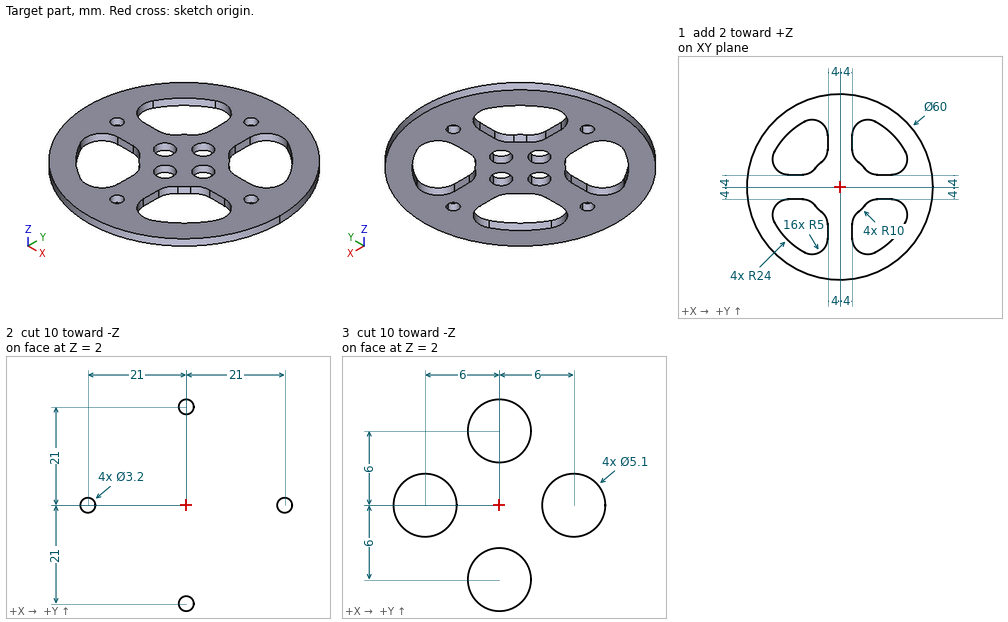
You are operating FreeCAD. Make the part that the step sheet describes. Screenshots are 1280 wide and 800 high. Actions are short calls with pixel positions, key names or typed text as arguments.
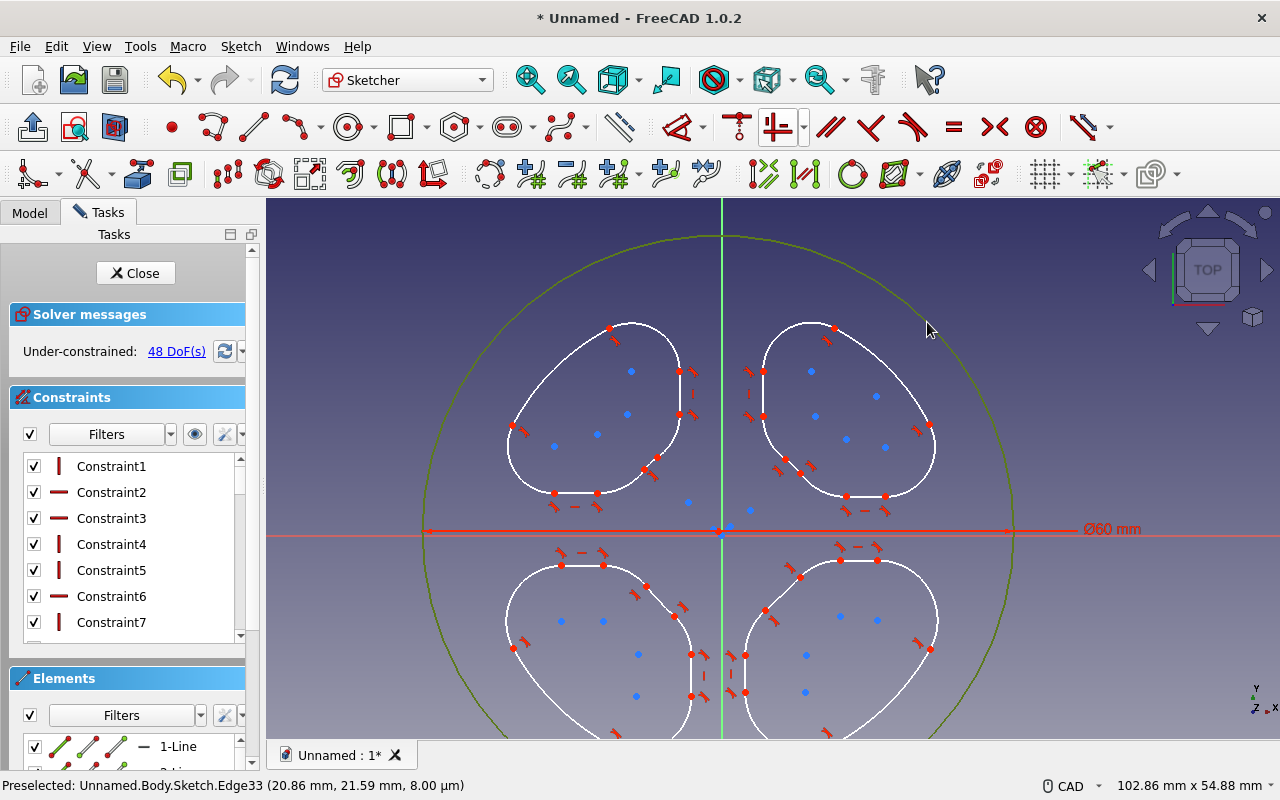
click(536, 683)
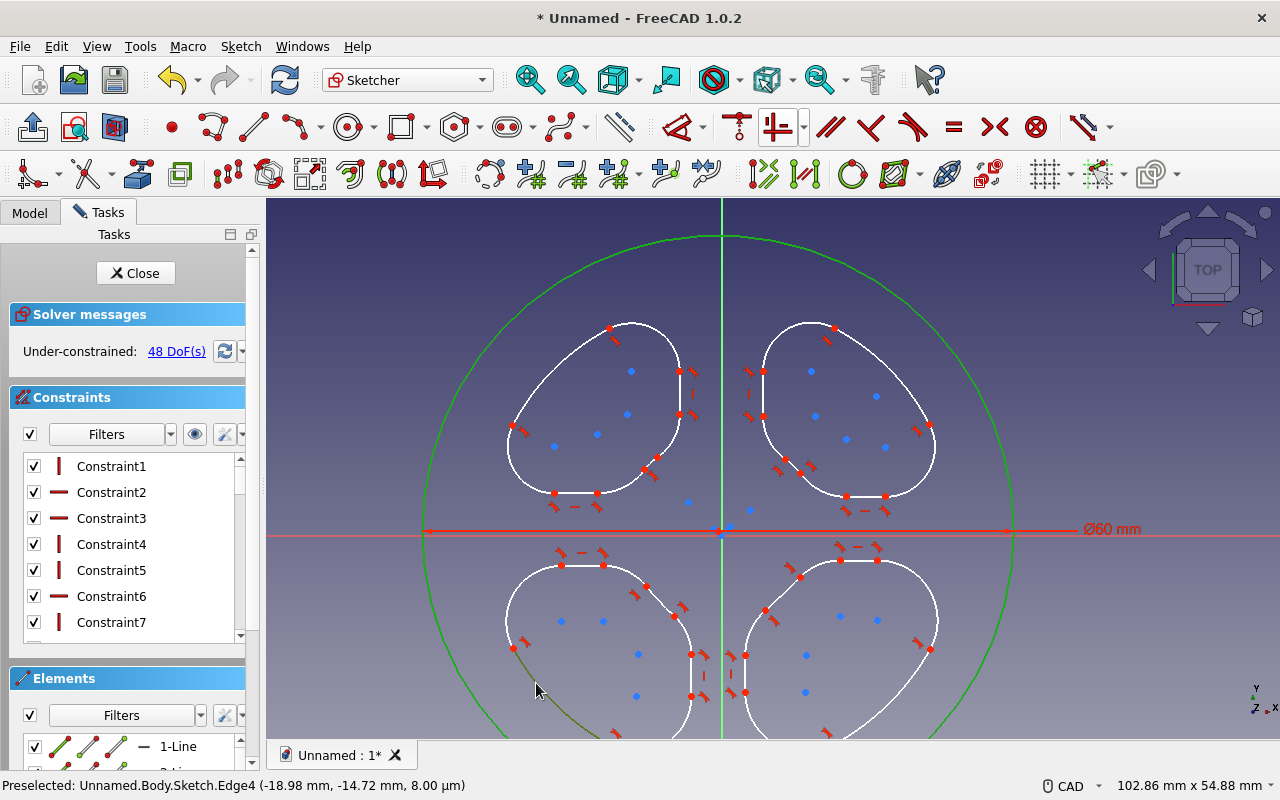
click(737, 128)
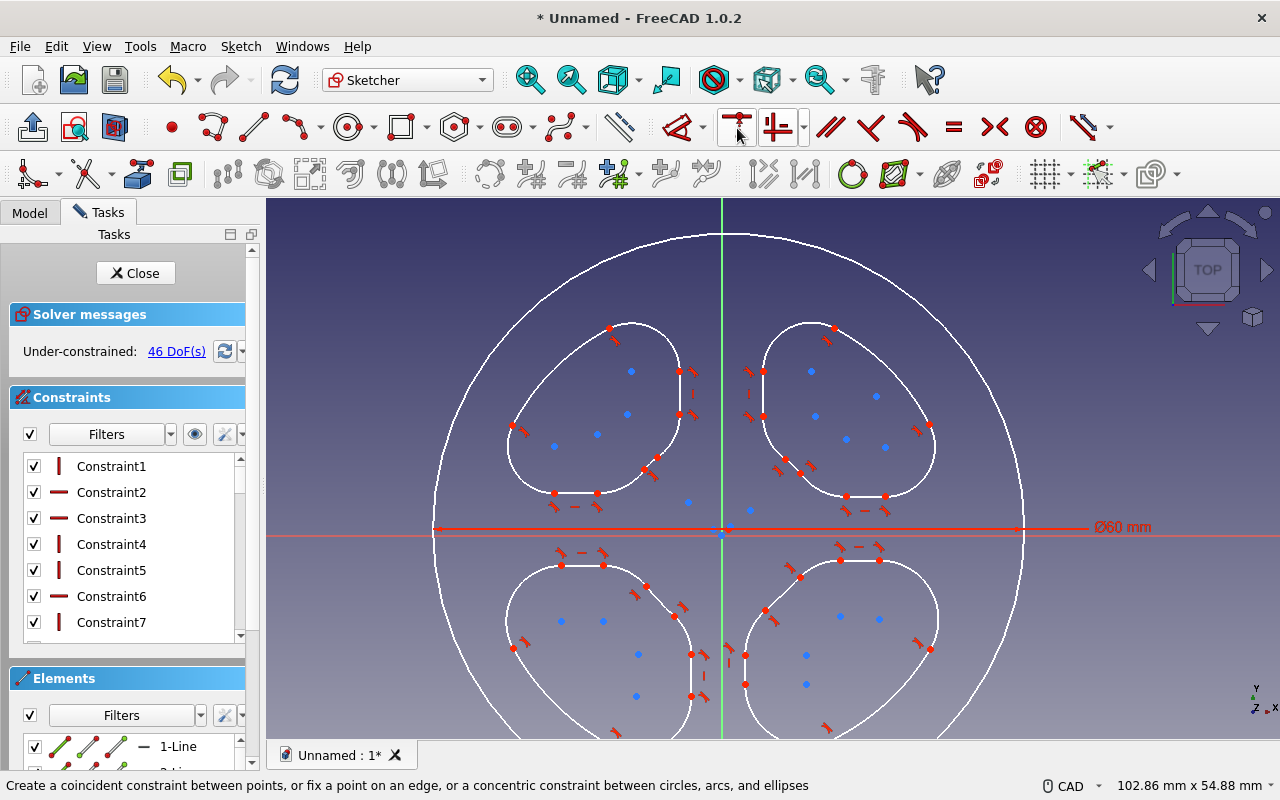
click(937, 320)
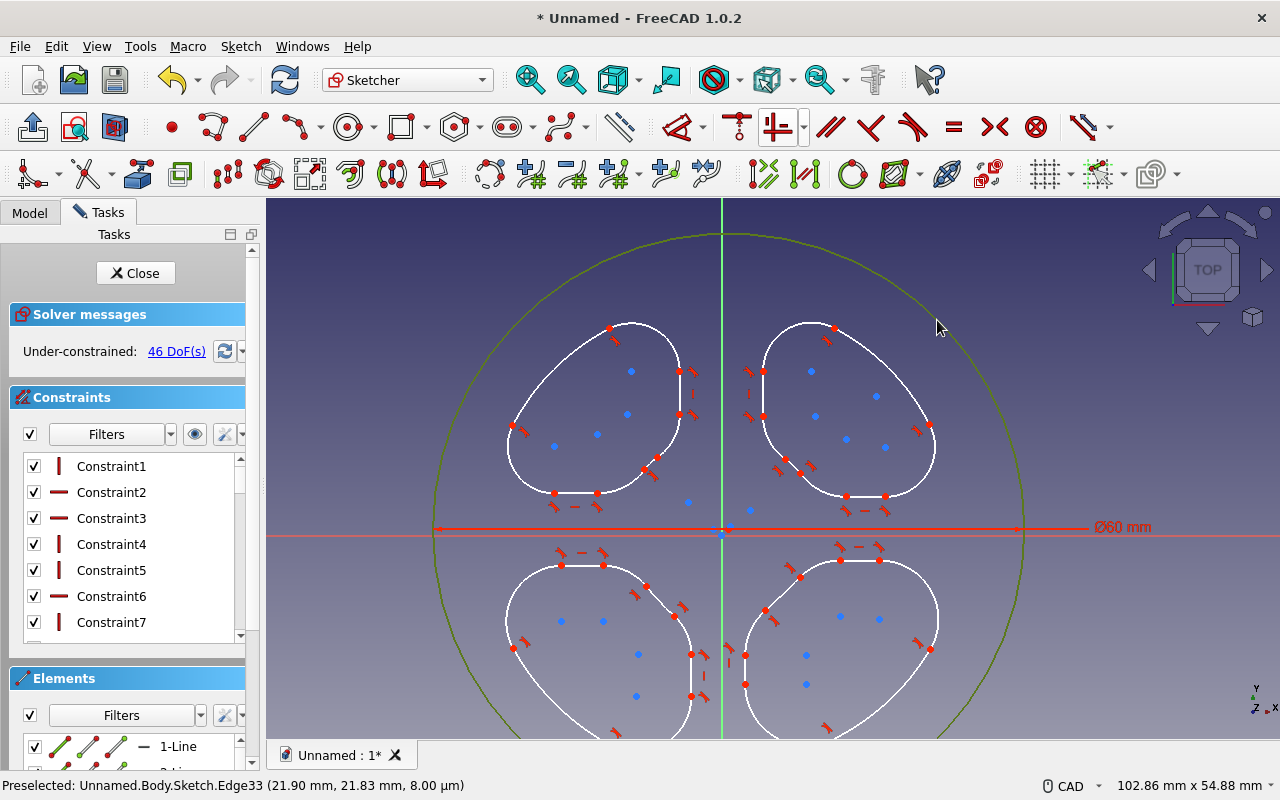
click(654, 596)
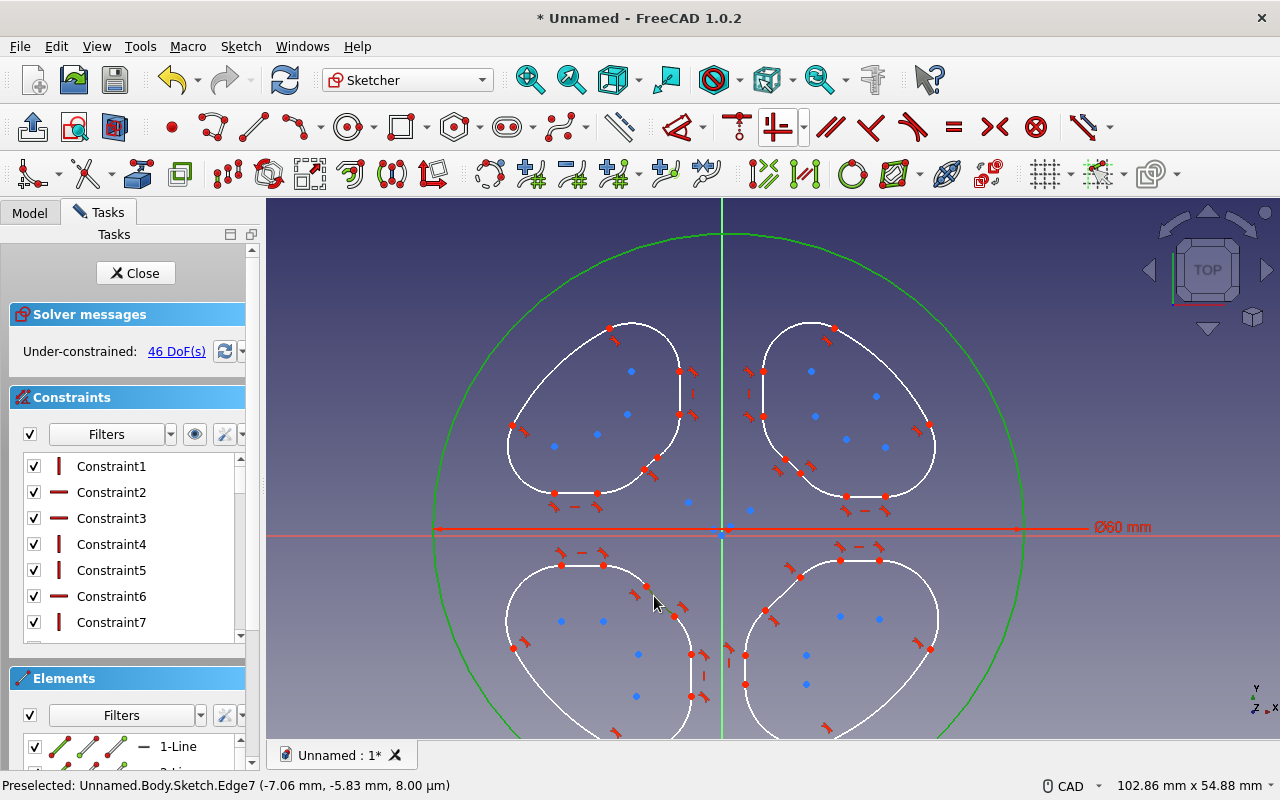
click(737, 128)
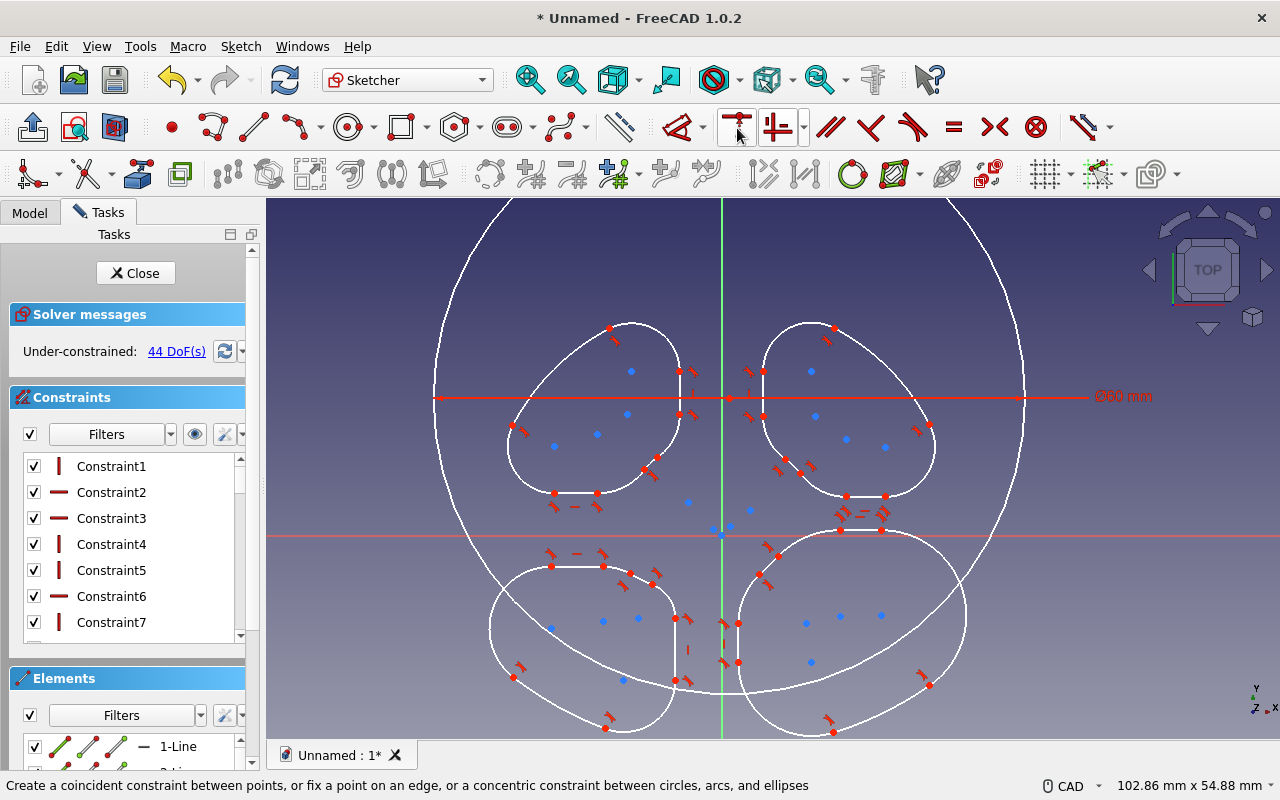
click(521, 608)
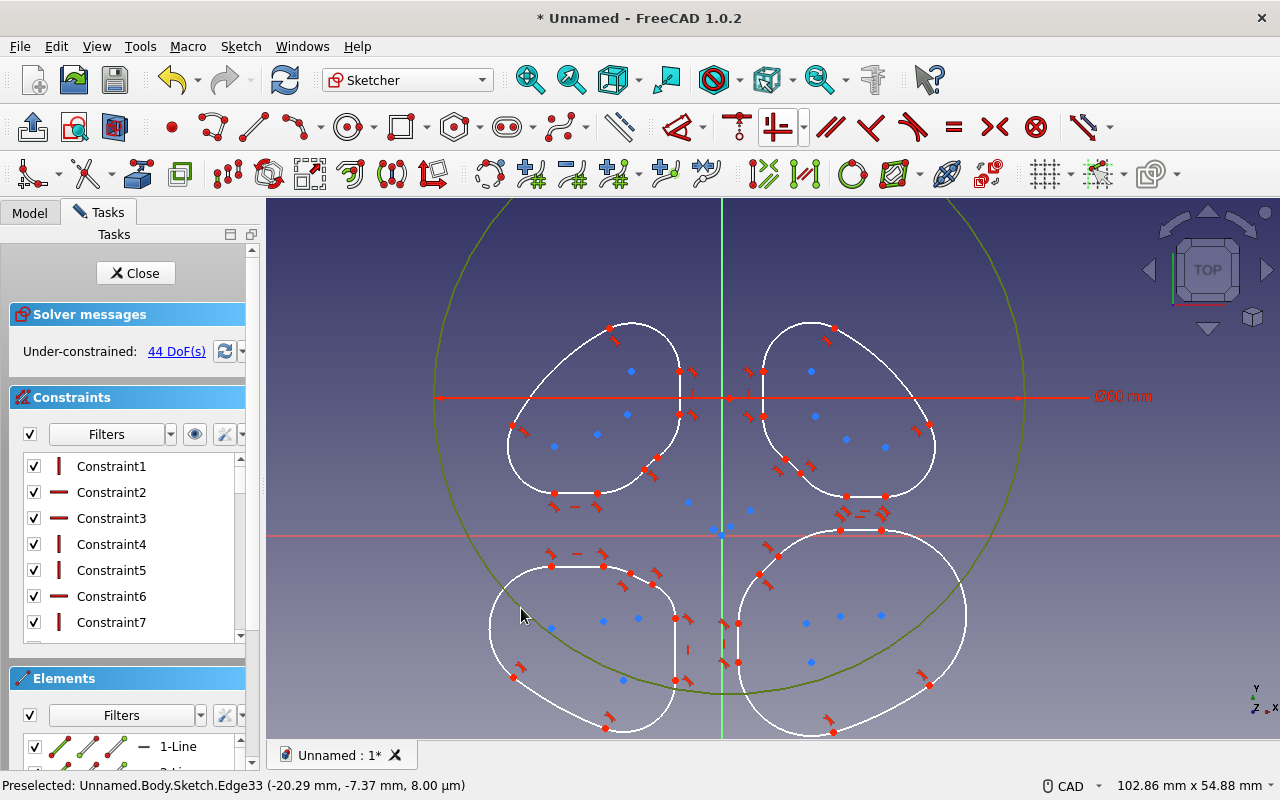
click(769, 565)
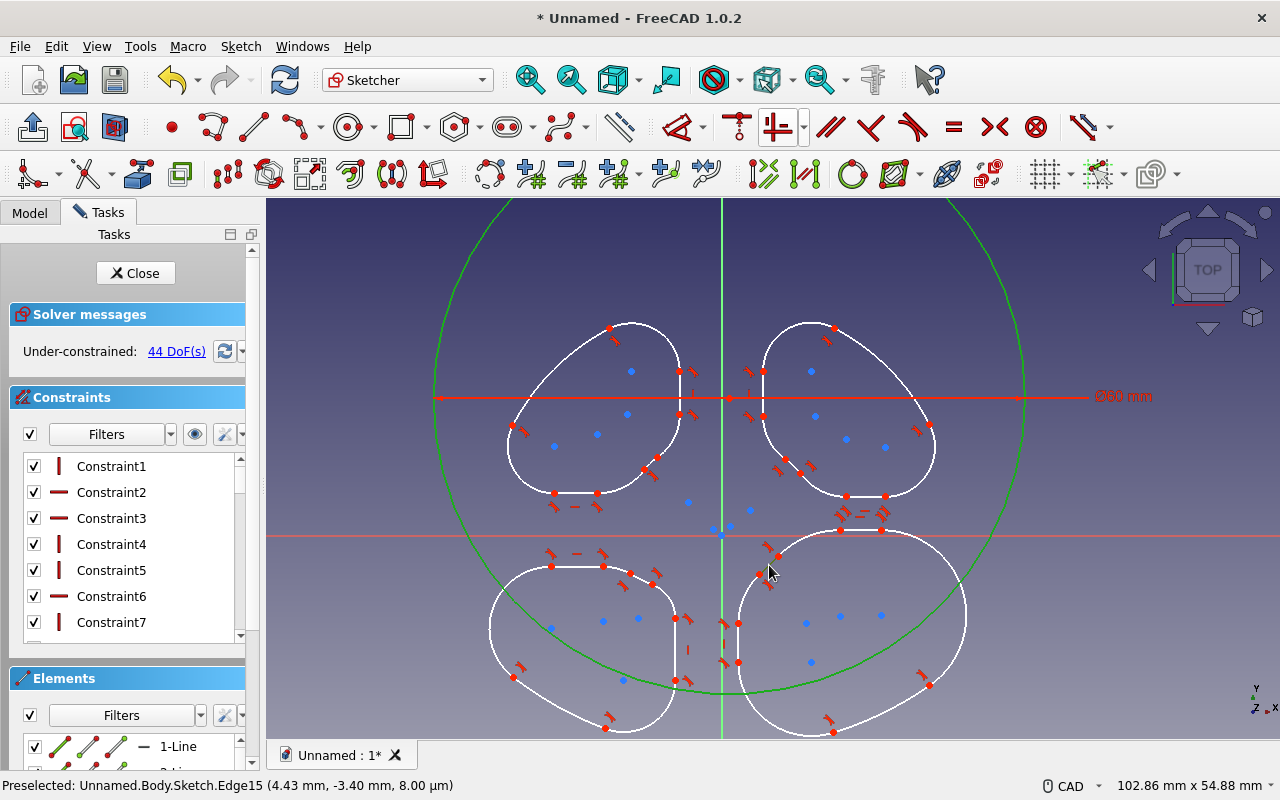
key(c)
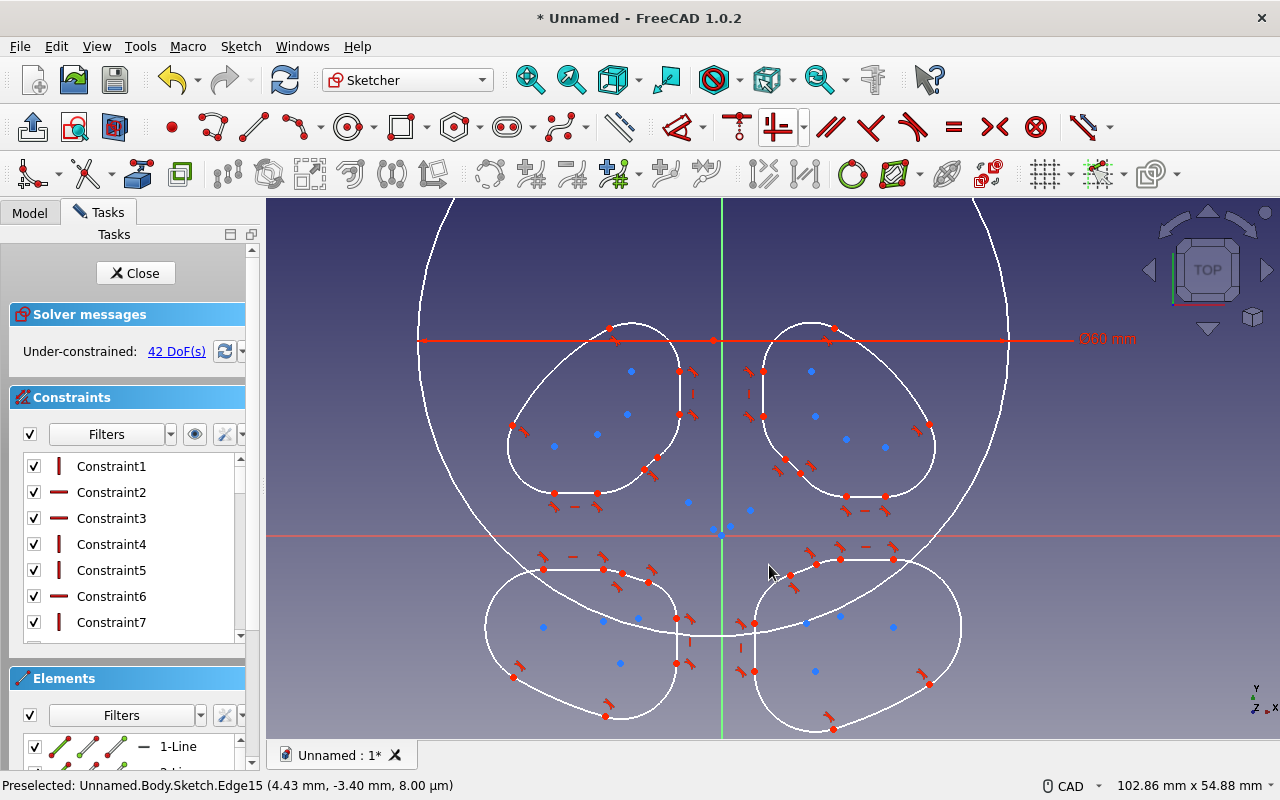
click(505, 551)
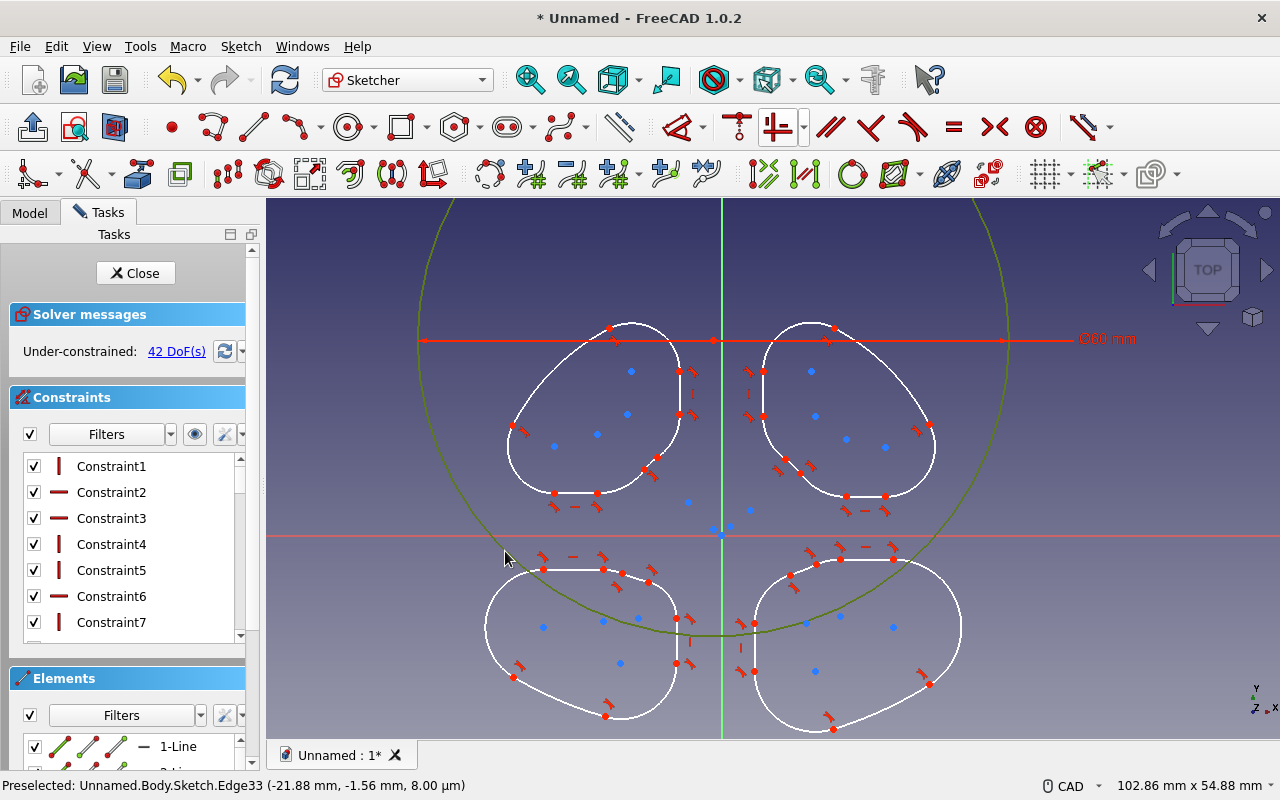
scroll(650, 463, up, 3)